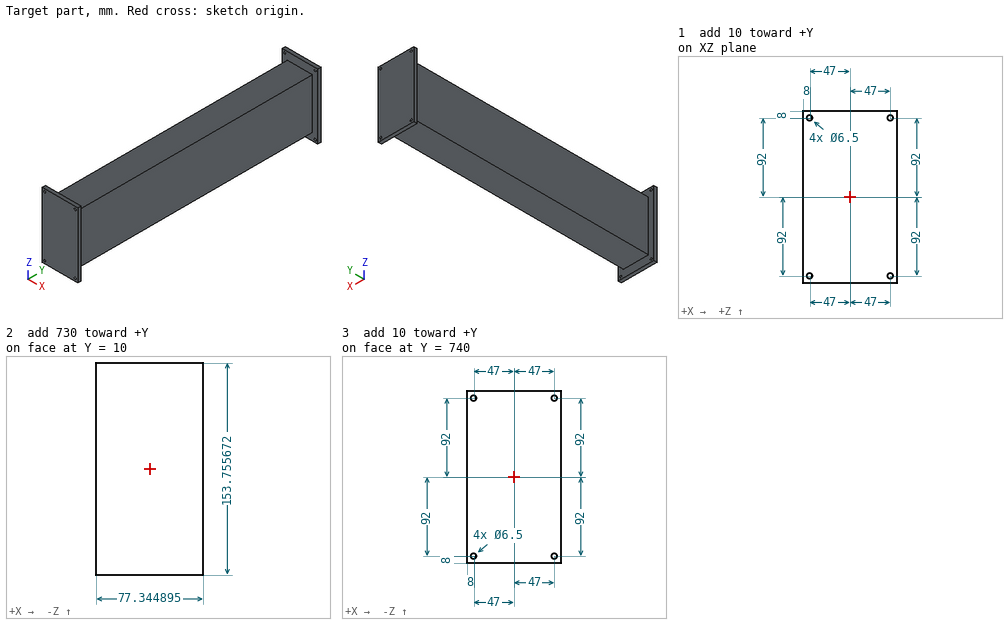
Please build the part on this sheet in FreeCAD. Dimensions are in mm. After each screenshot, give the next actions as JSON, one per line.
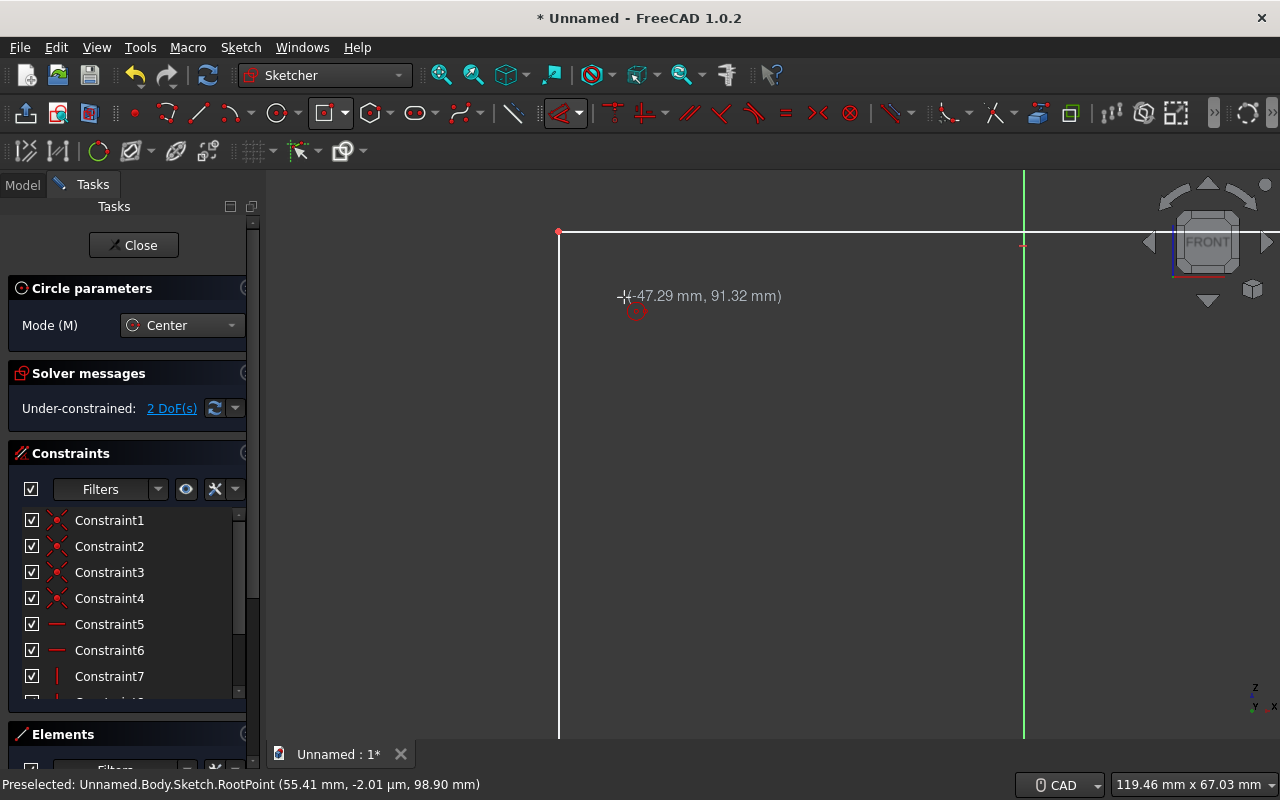
{"action": "scroll", "coordinate": [624, 297], "scroll_direction": "down", "scroll_amount": 8}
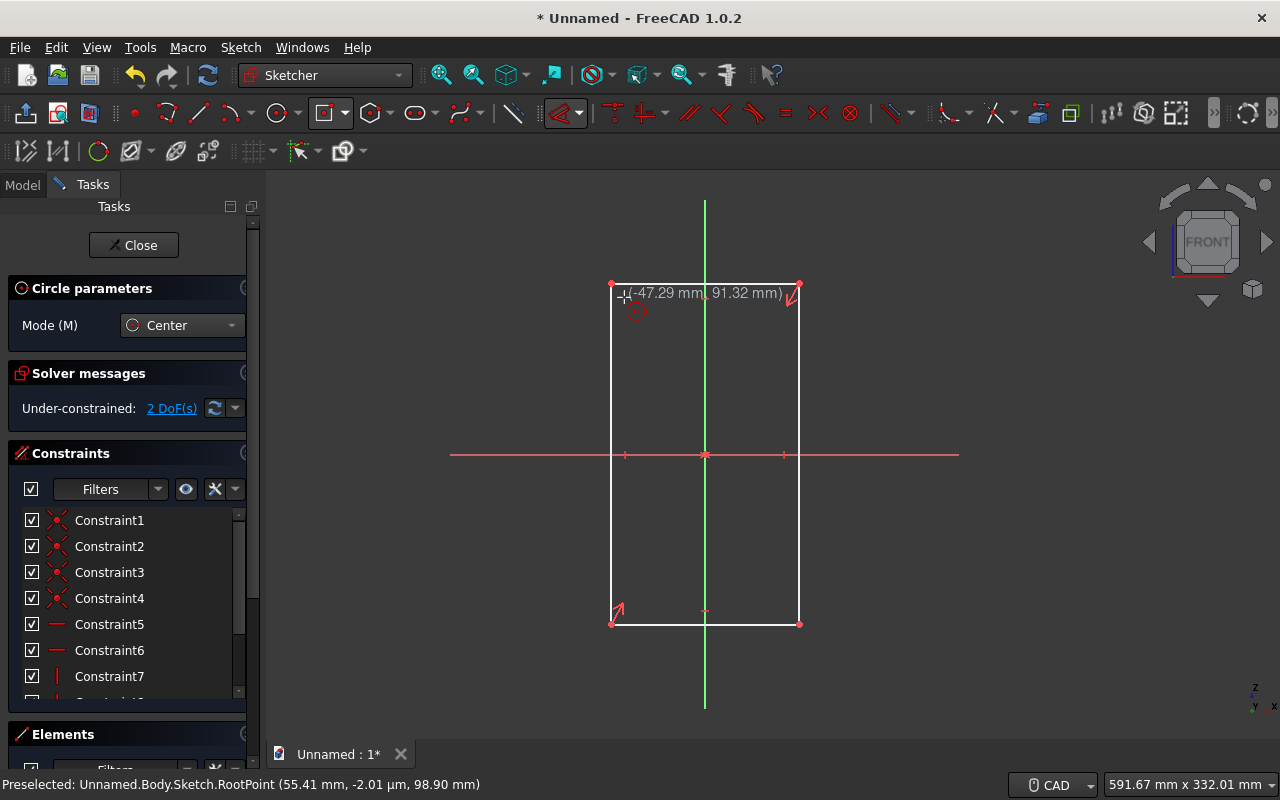
{"action": "left_click", "coordinate": [624, 297]}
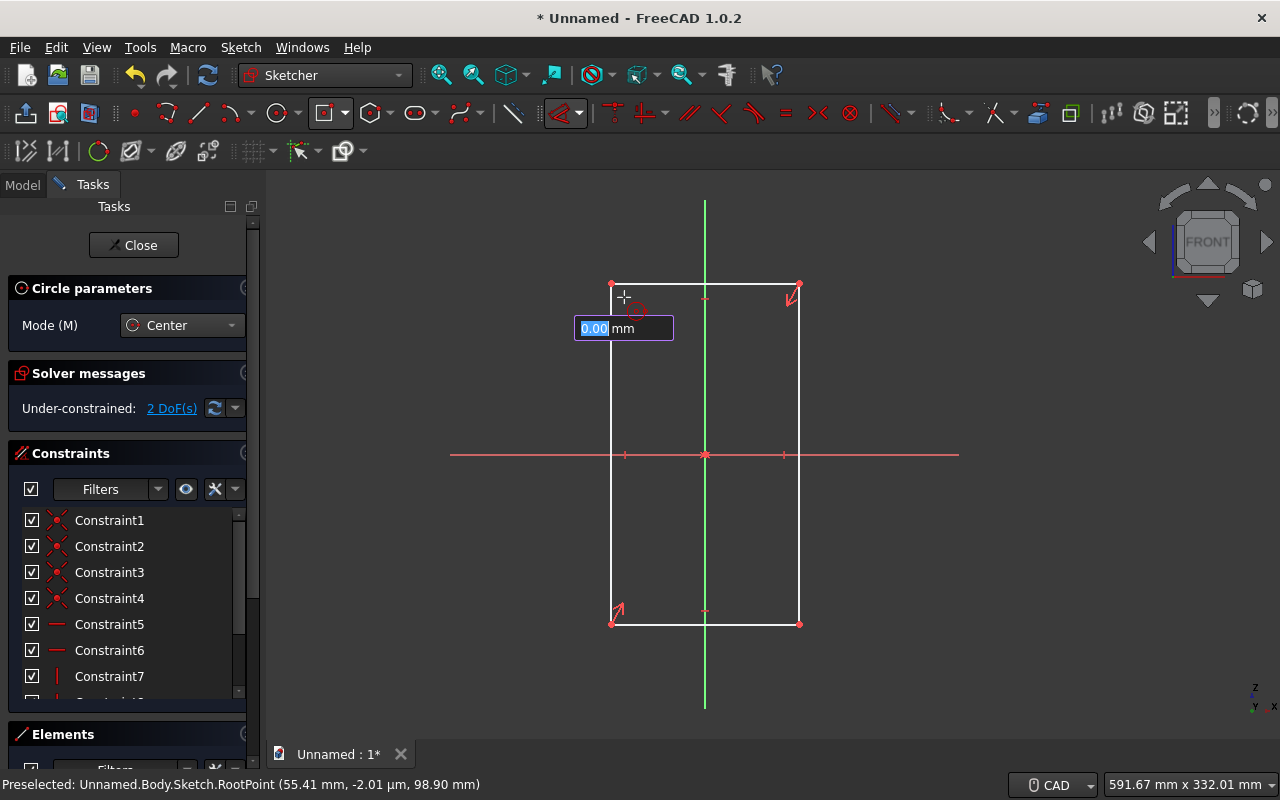
{"action": "scroll", "coordinate": [628, 301], "scroll_direction": "up", "scroll_amount": 6}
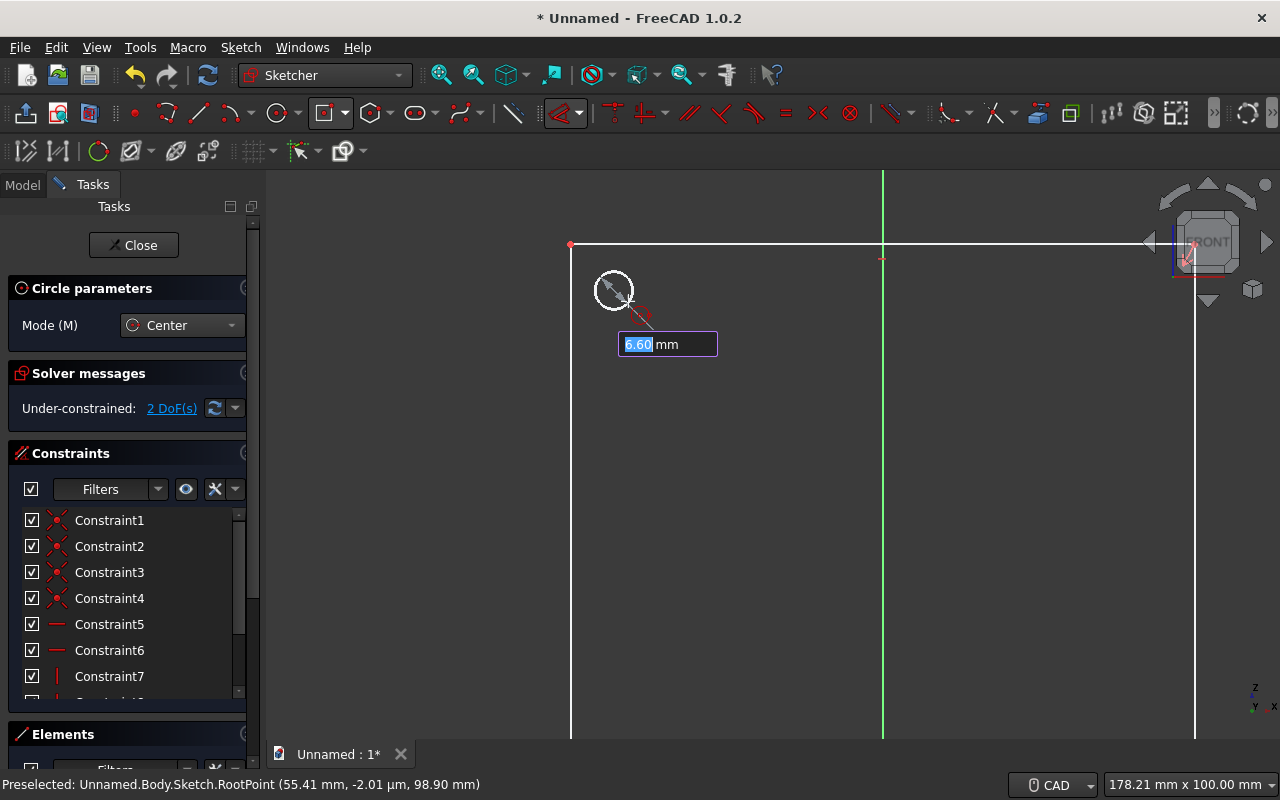
{"action": "left_click", "coordinate": [629, 300]}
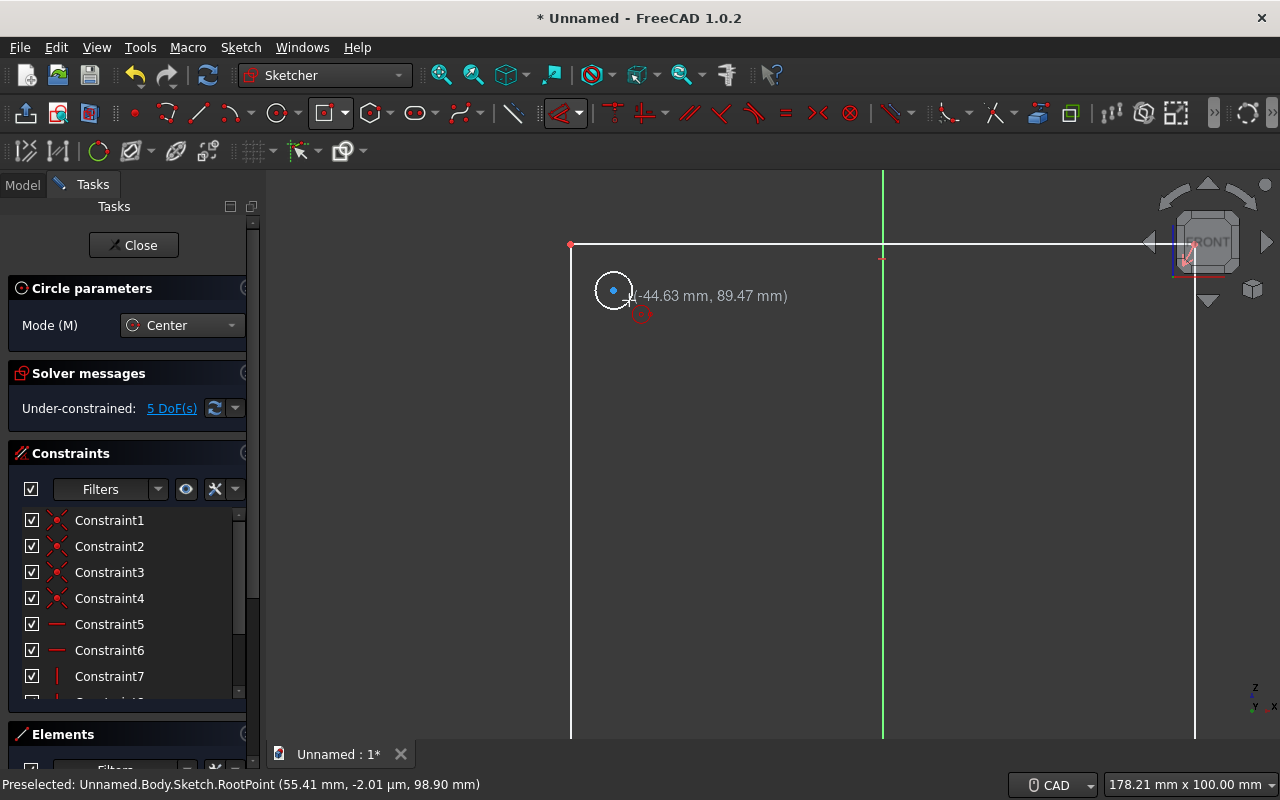
{"action": "scroll", "coordinate": [628, 301], "scroll_direction": "down", "scroll_amount": 6}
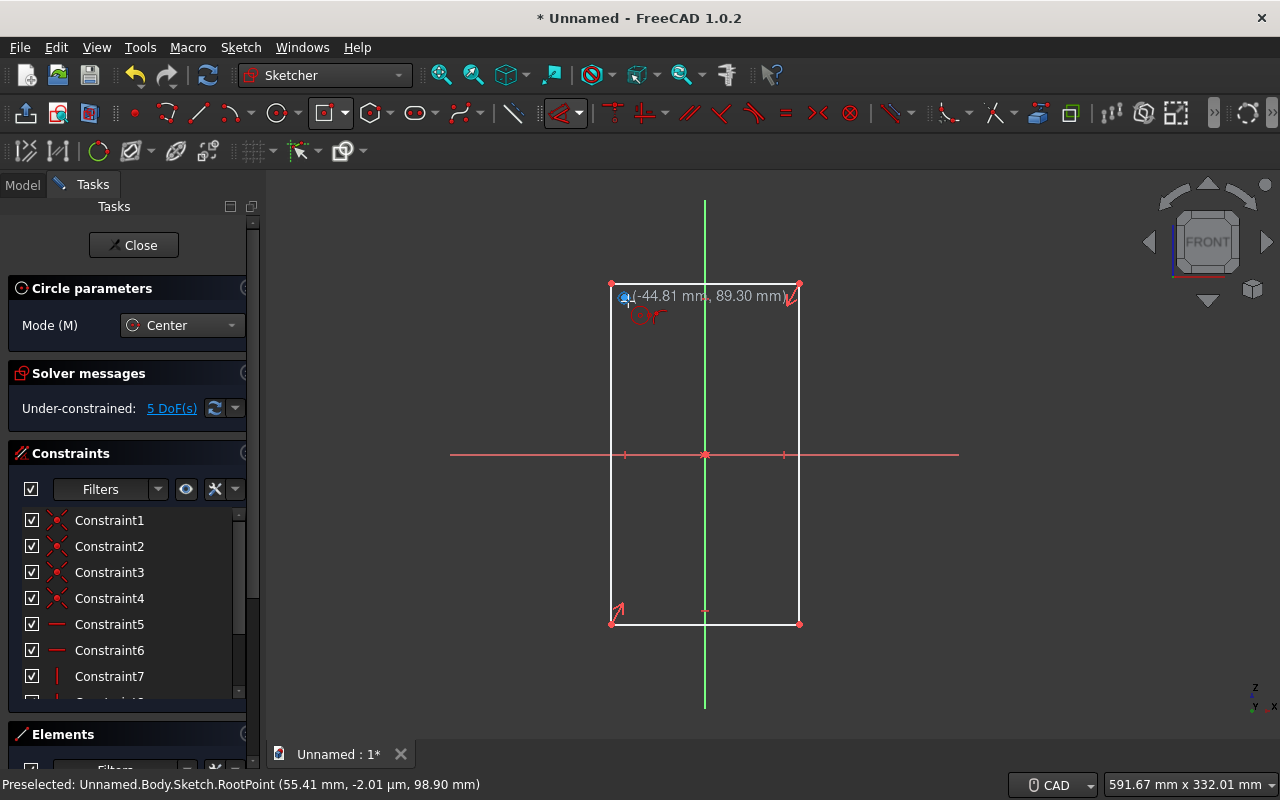
{"action": "scroll", "coordinate": [786, 297], "scroll_direction": "up", "scroll_amount": 8}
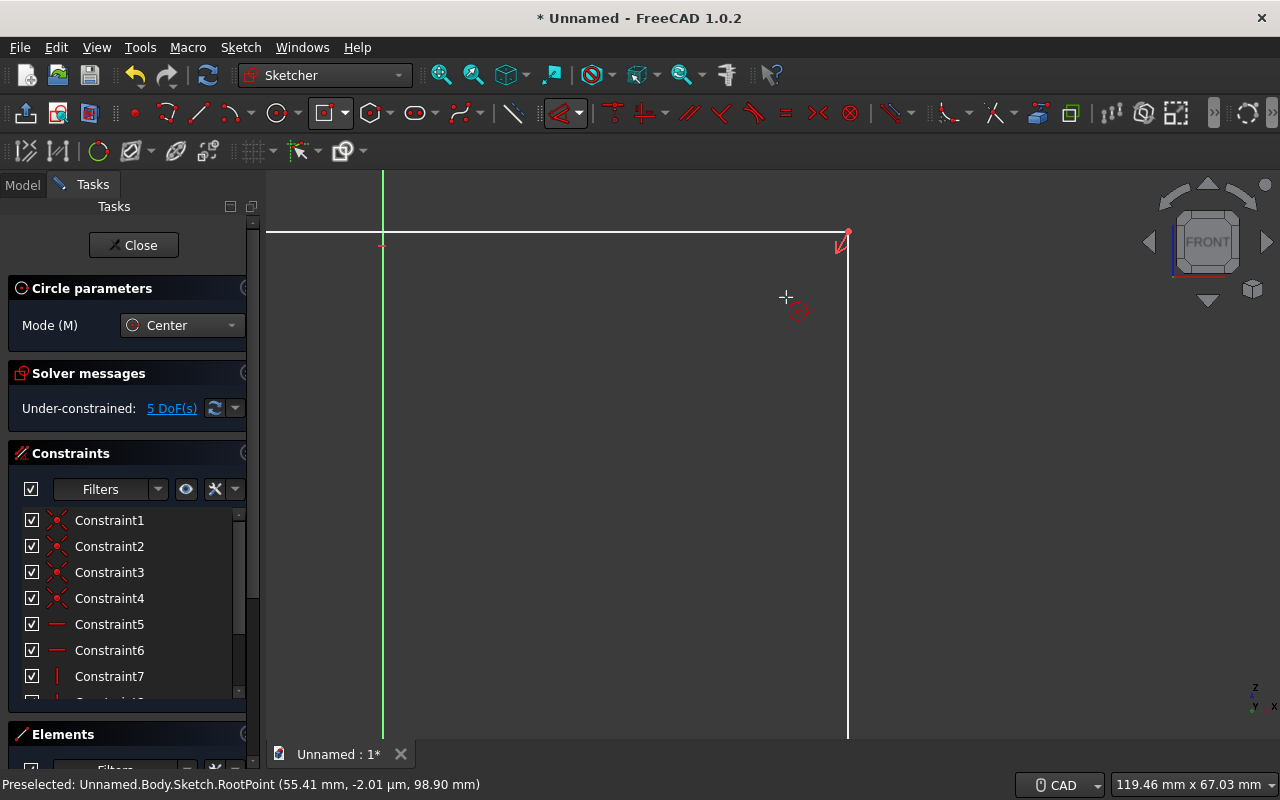
{"action": "scroll", "coordinate": [786, 297], "scroll_direction": "down", "scroll_amount": 8}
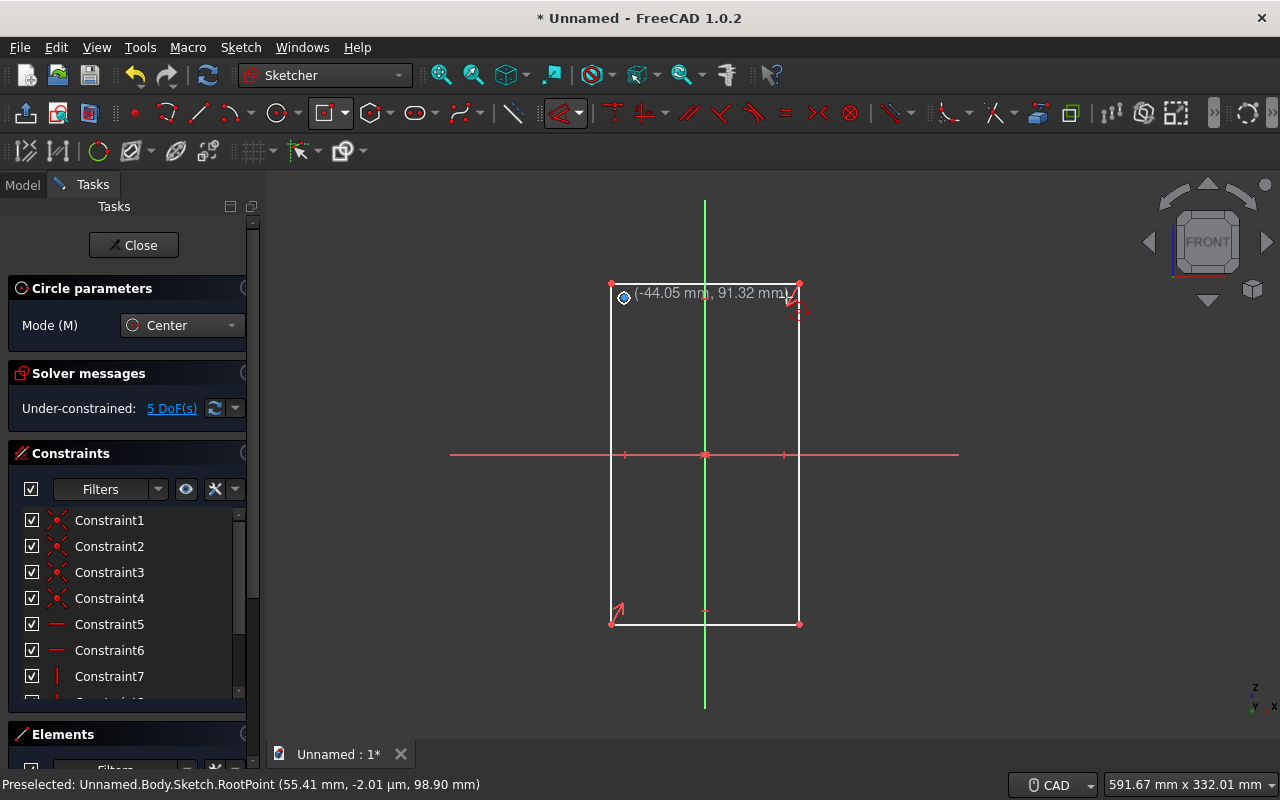
{"action": "left_click", "coordinate": [786, 297]}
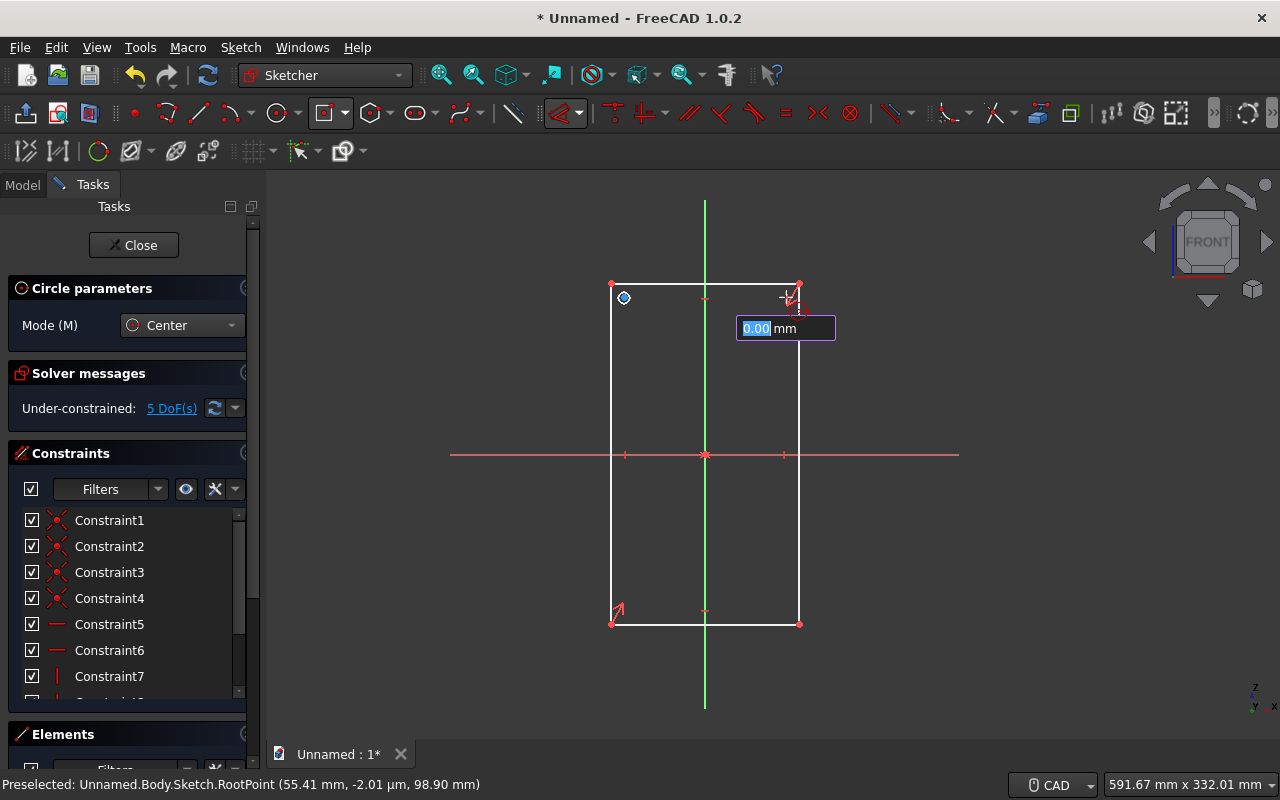
{"action": "scroll", "coordinate": [782, 301], "scroll_direction": "up", "scroll_amount": 6}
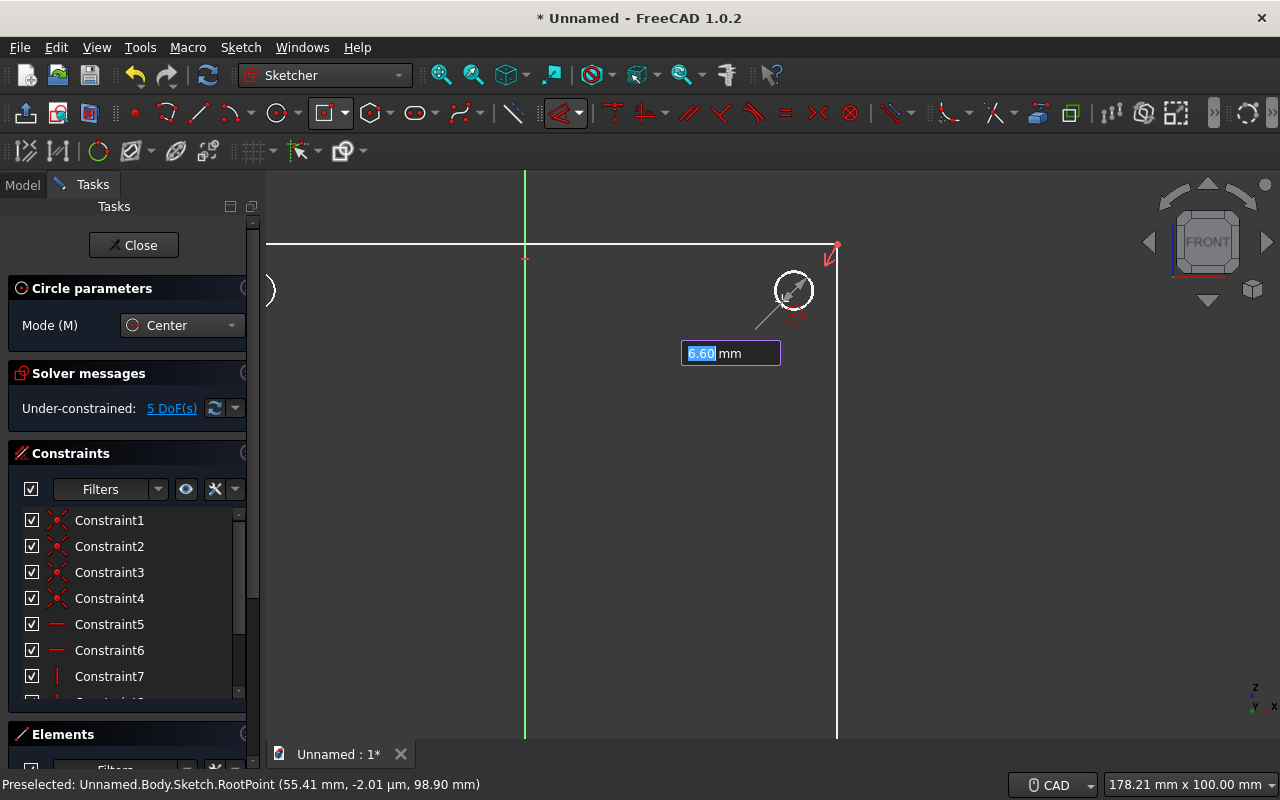
{"action": "left_click", "coordinate": [780, 300]}